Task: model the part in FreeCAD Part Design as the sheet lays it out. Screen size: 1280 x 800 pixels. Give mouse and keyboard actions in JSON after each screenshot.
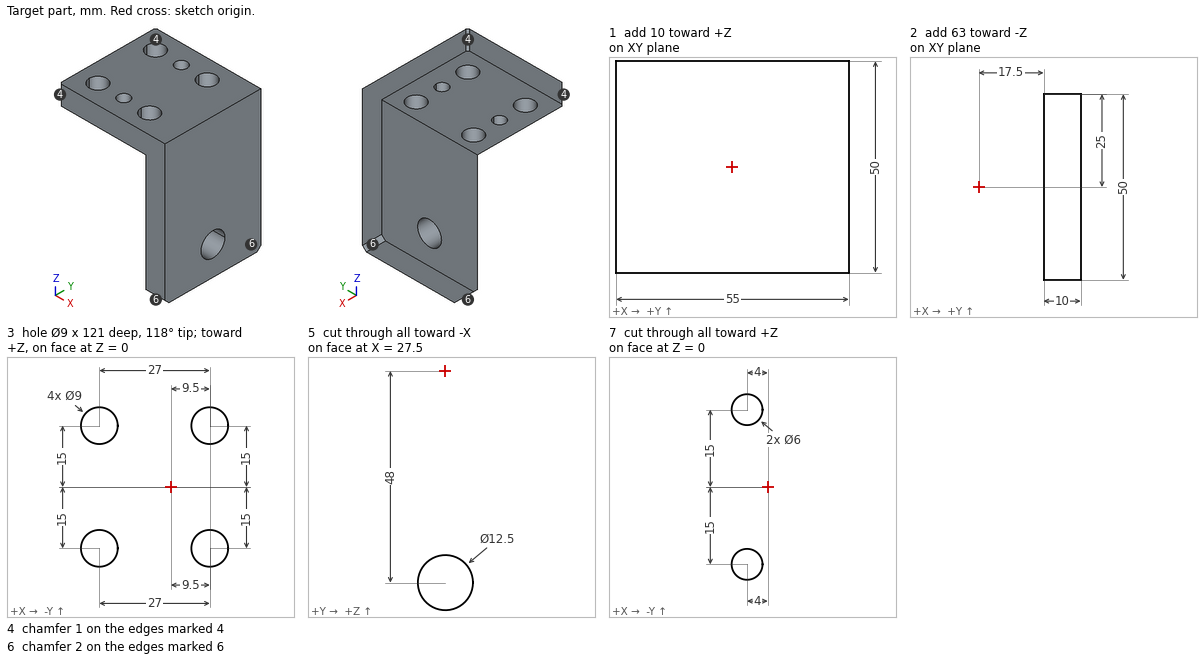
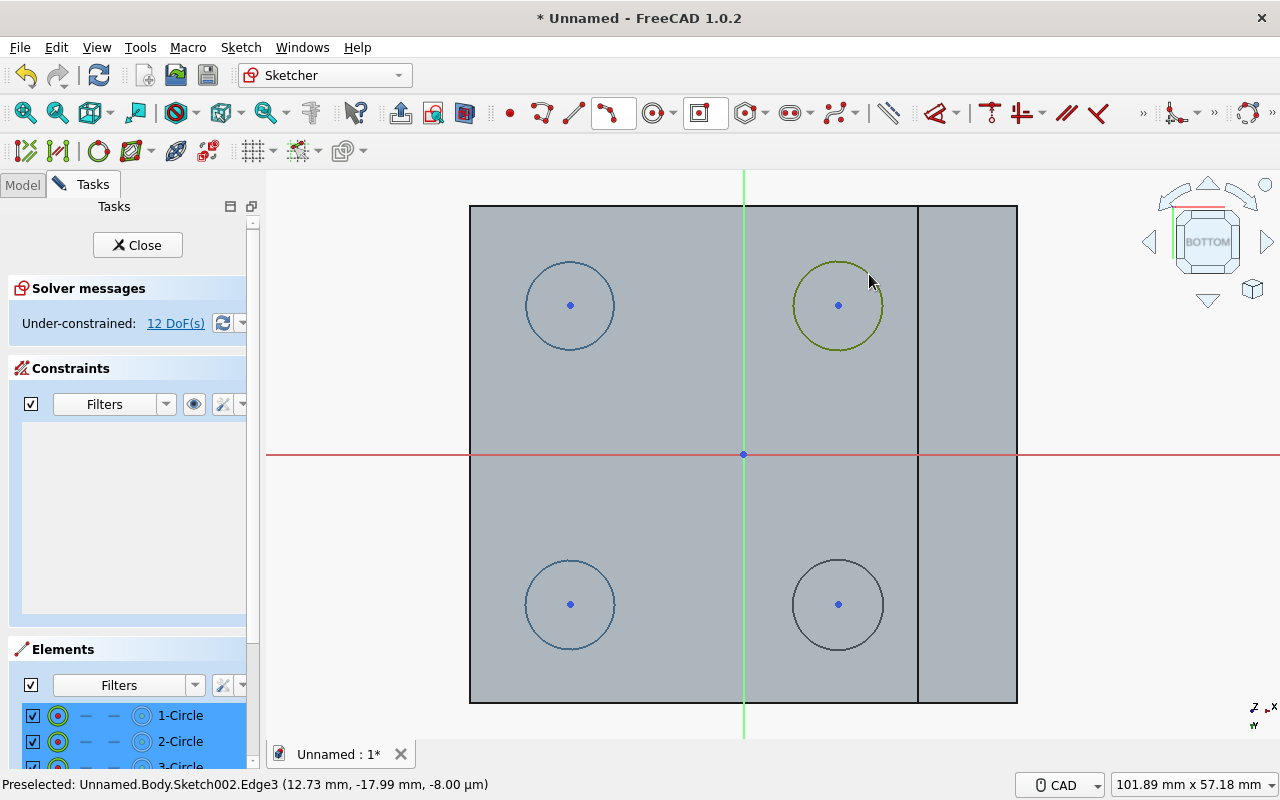
{"action": "left_click", "coordinate": [870, 573]}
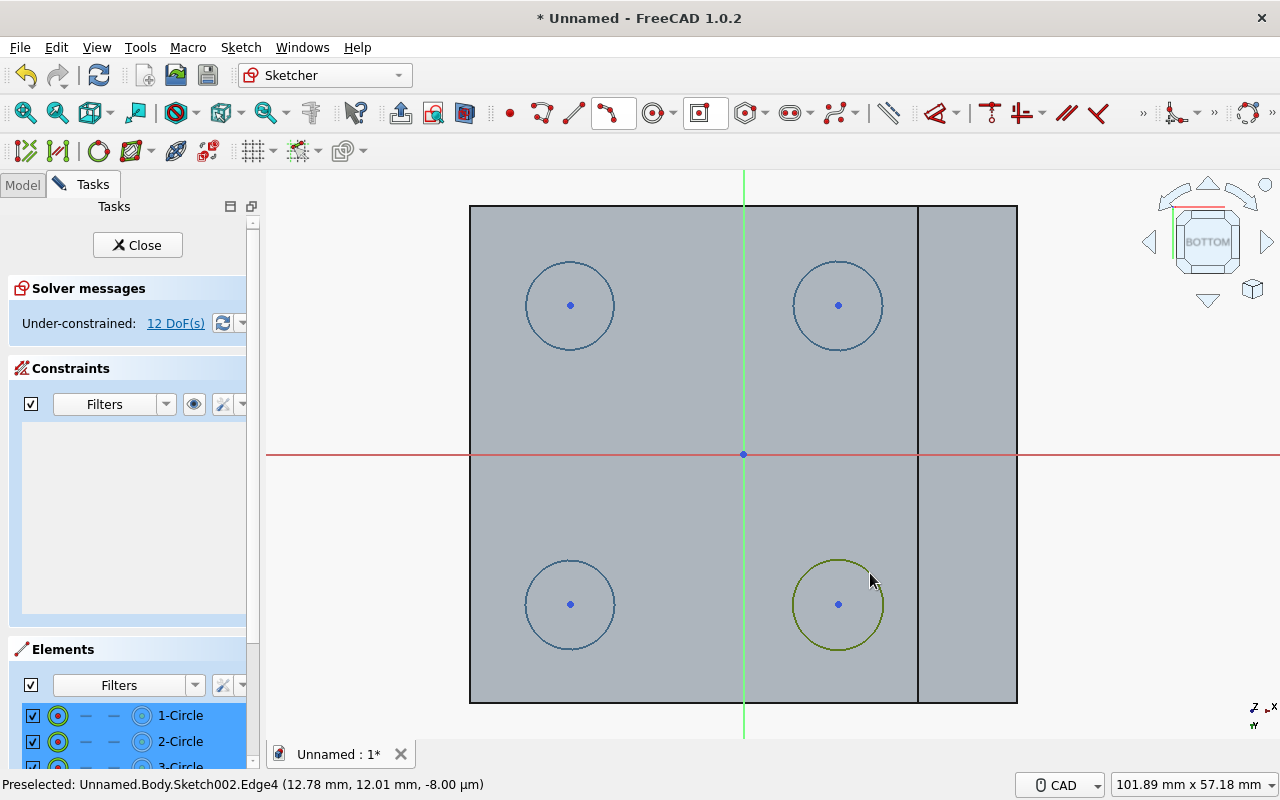
{"action": "key", "text": "e"}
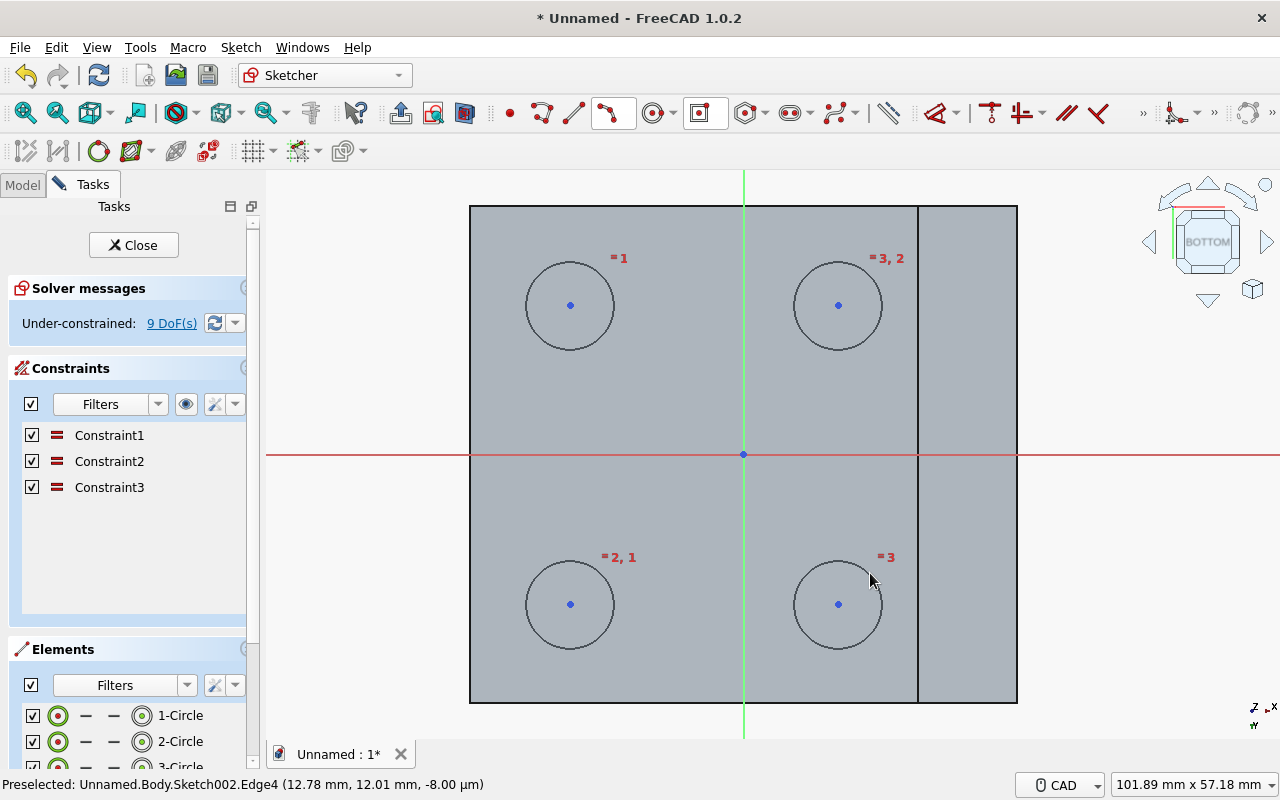
{"action": "key", "text": "d"}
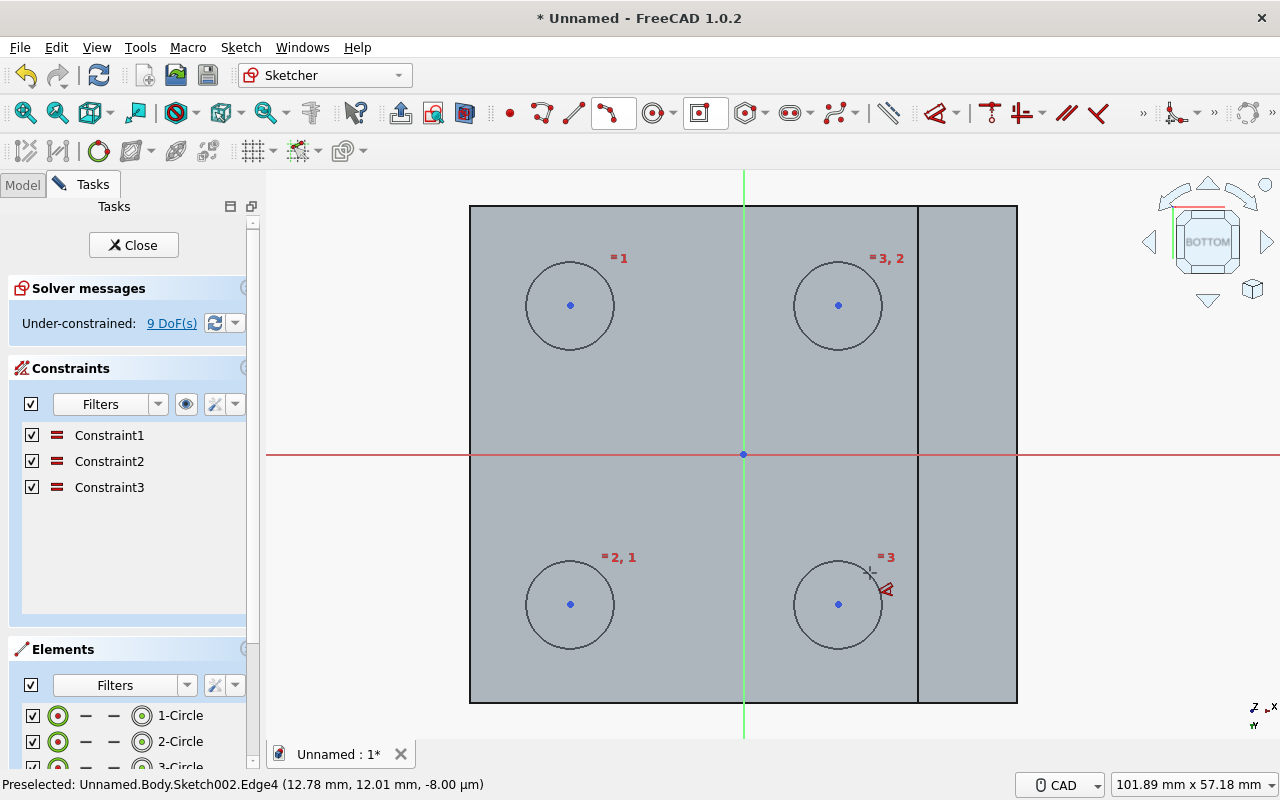
{"action": "left_click", "coordinate": [601, 275]}
{"action": "left_click", "coordinate": [624, 252]}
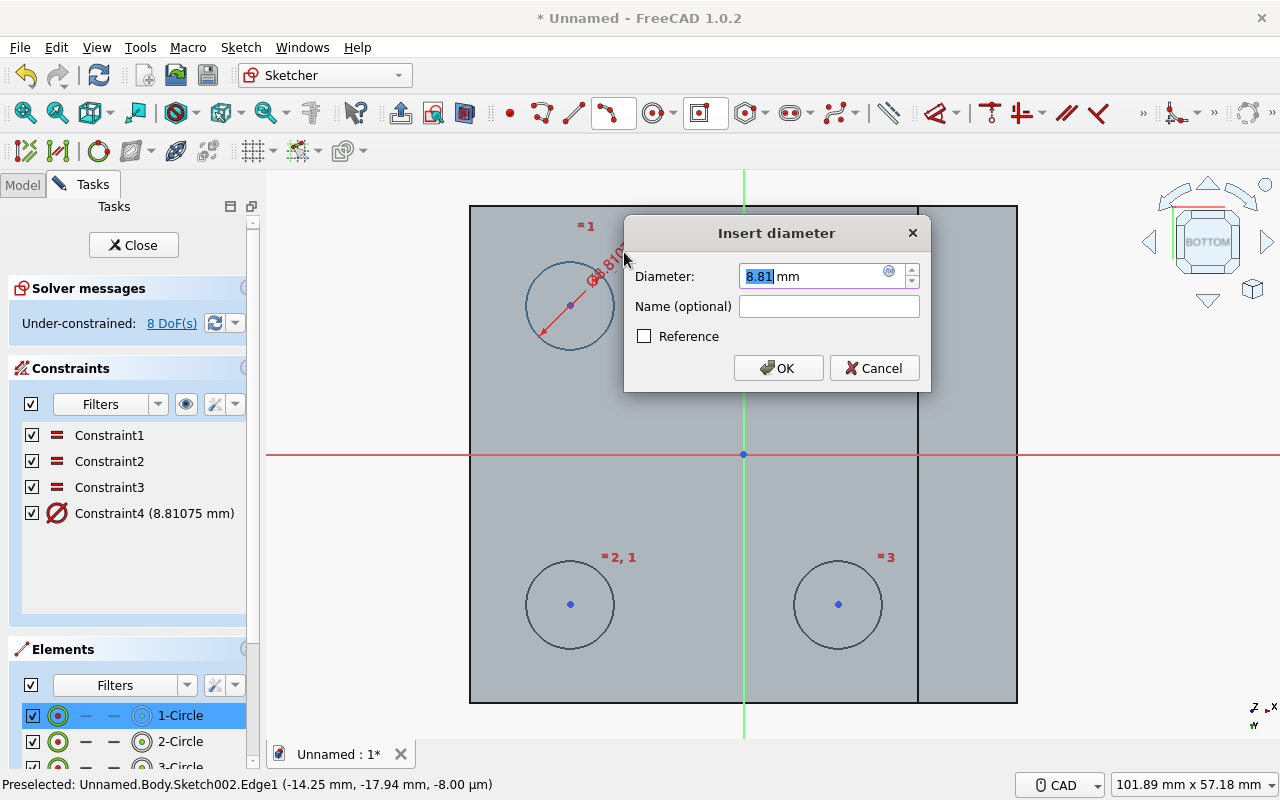
{"action": "type", "text": "9"}
{"action": "key", "text": "Return"}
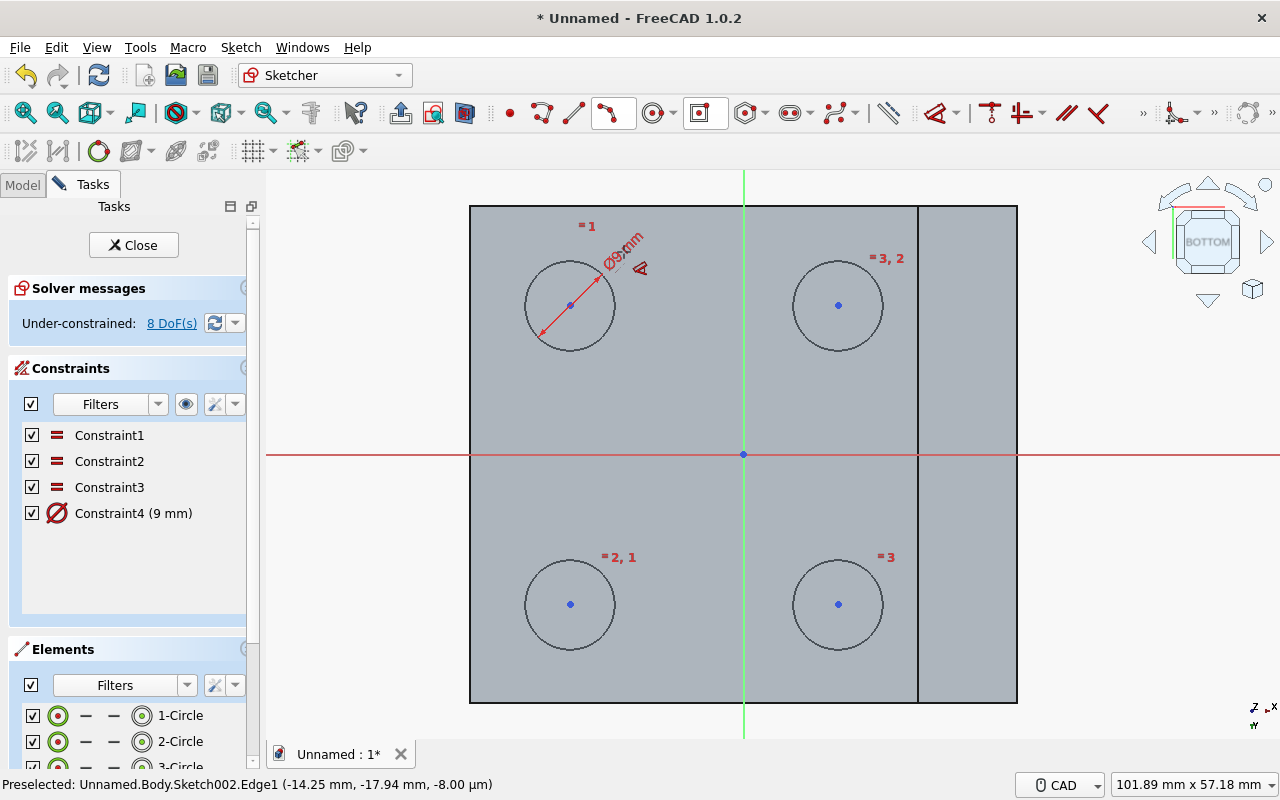
{"action": "left_click", "coordinate": [570, 306]}
{"action": "left_click", "coordinate": [536, 380]}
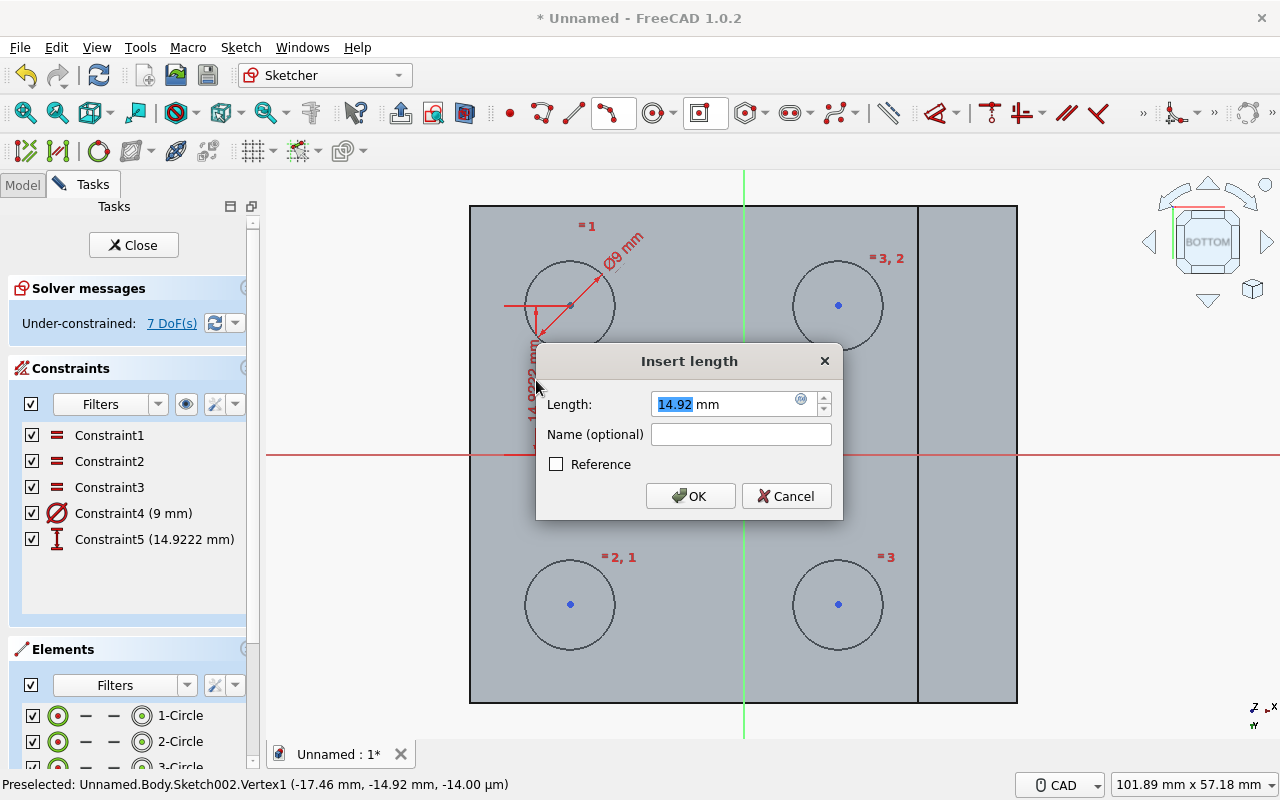
{"action": "type", "text": "15"}
{"action": "key", "text": "Return"}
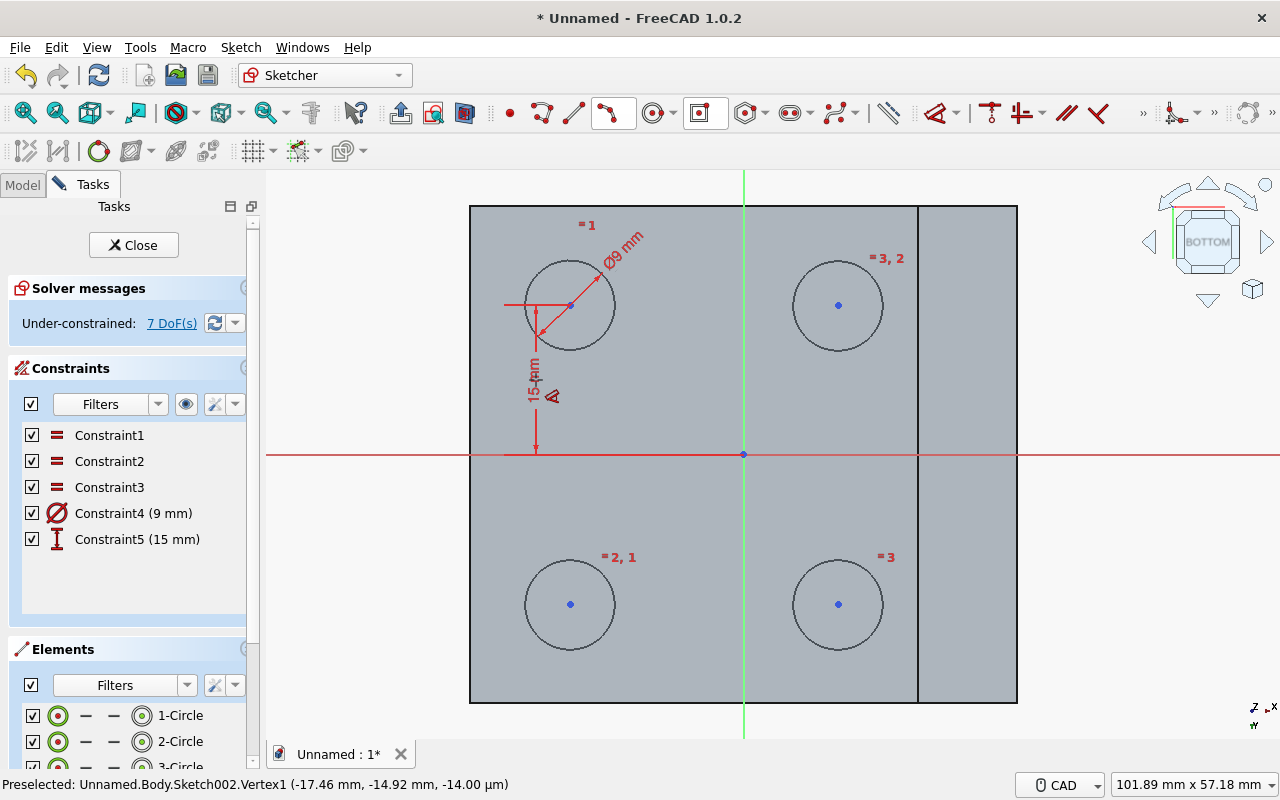
{"action": "left_click", "coordinate": [570, 605]}
{"action": "left_click", "coordinate": [536, 530]}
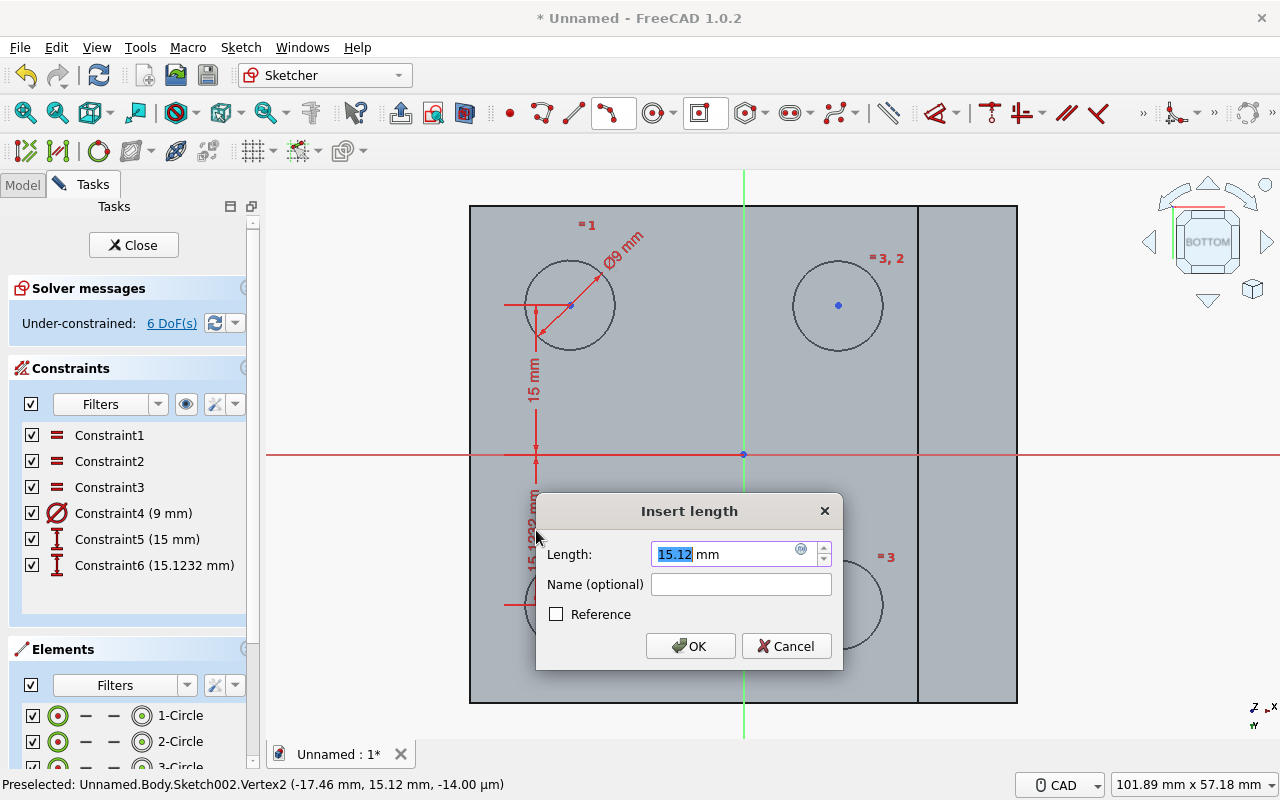
{"action": "type", "text": "15"}
{"action": "key", "text": "Return"}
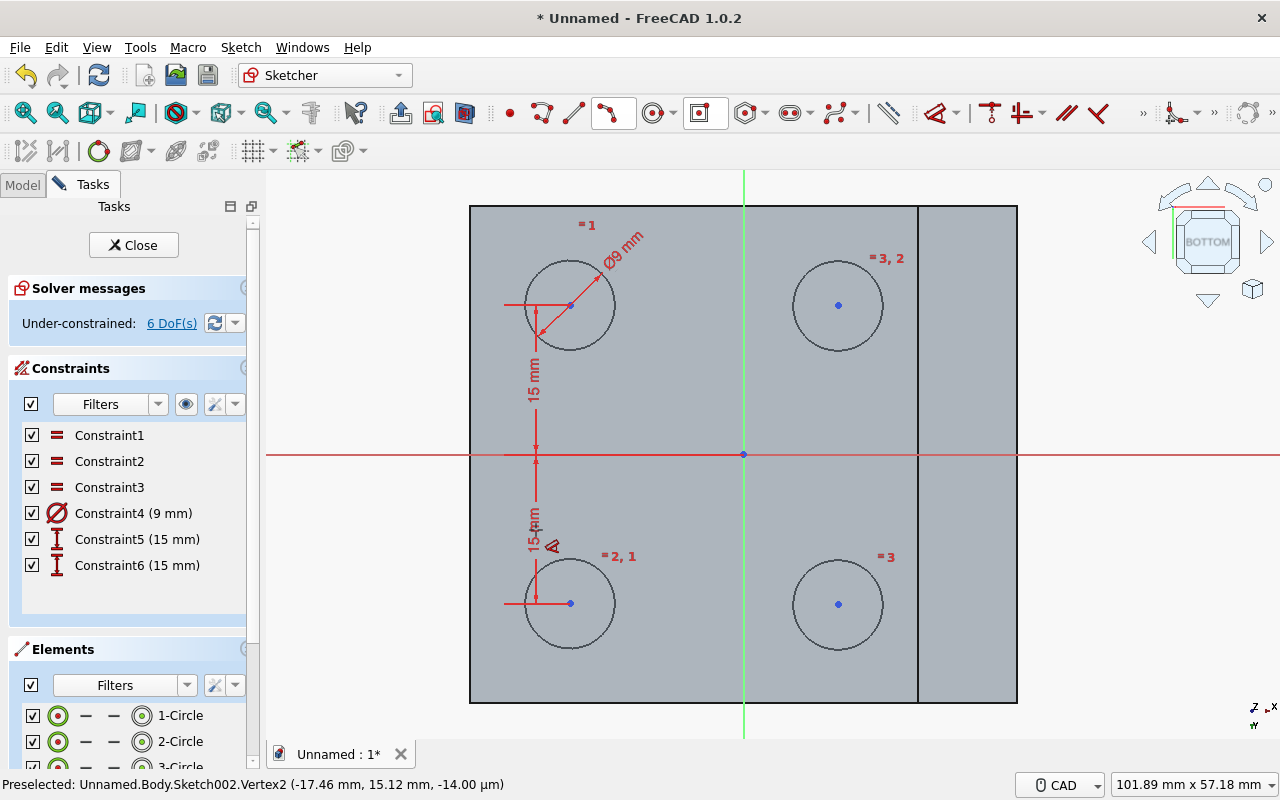
{"action": "left_click", "coordinate": [838, 306]}
{"action": "left_click", "coordinate": [872, 380]}